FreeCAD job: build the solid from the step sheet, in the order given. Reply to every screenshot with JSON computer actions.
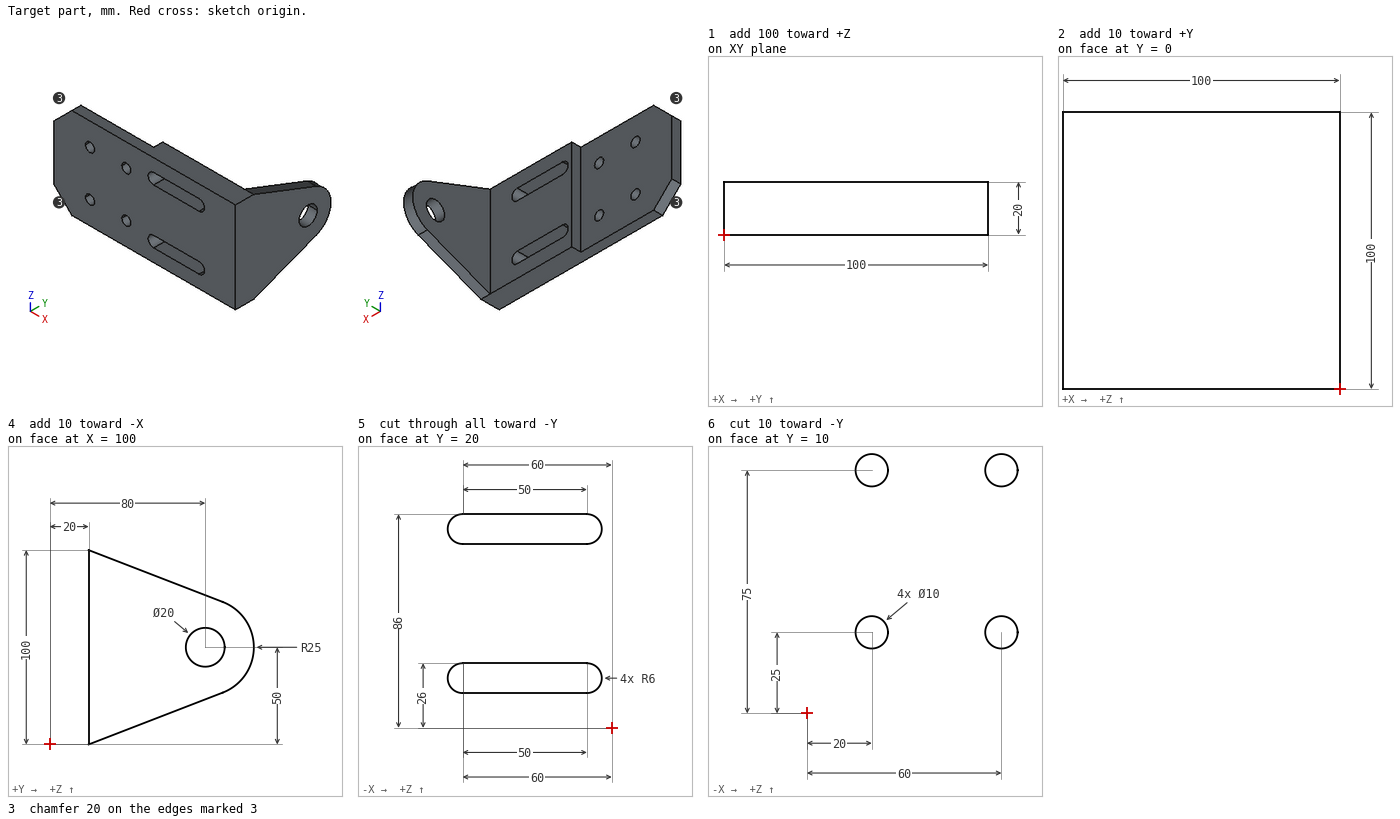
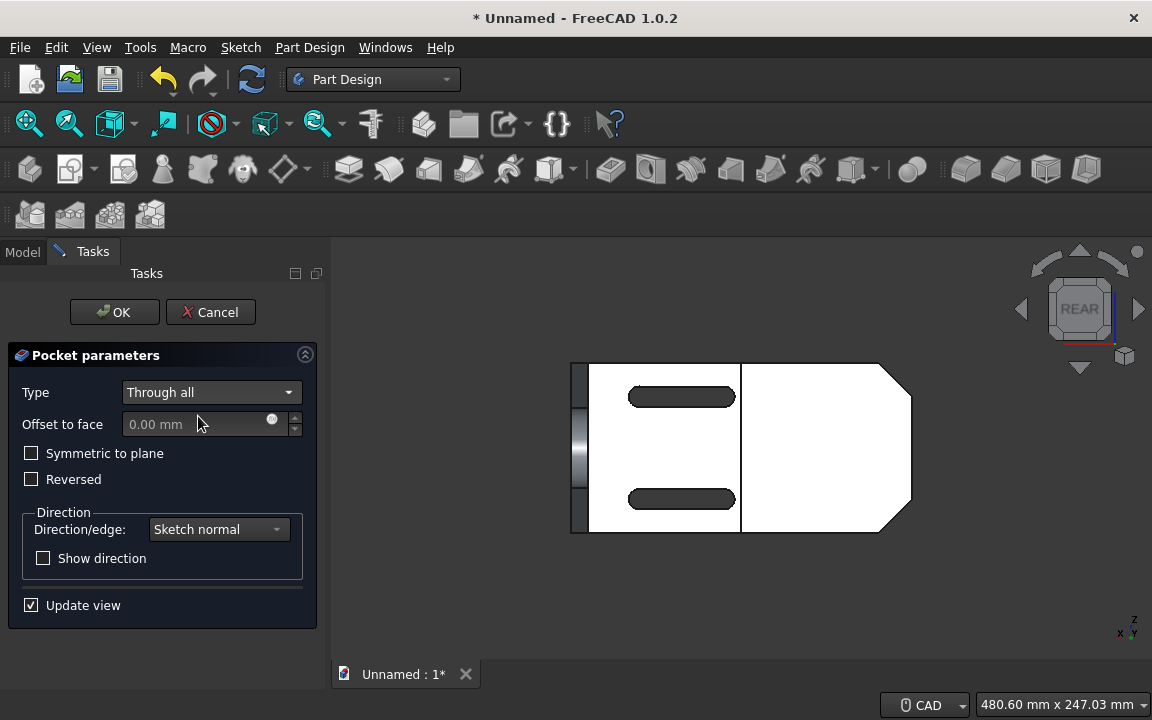
{"action": "left_click", "coordinate": [115, 312]}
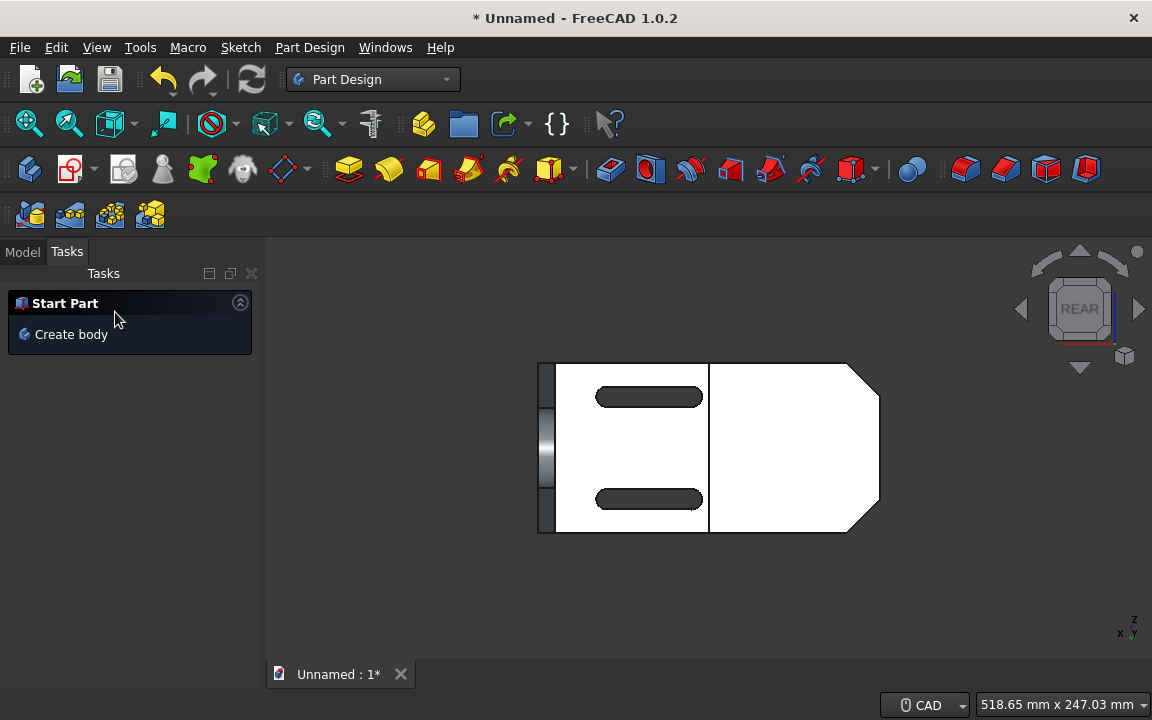
{"action": "left_click", "coordinate": [30, 124]}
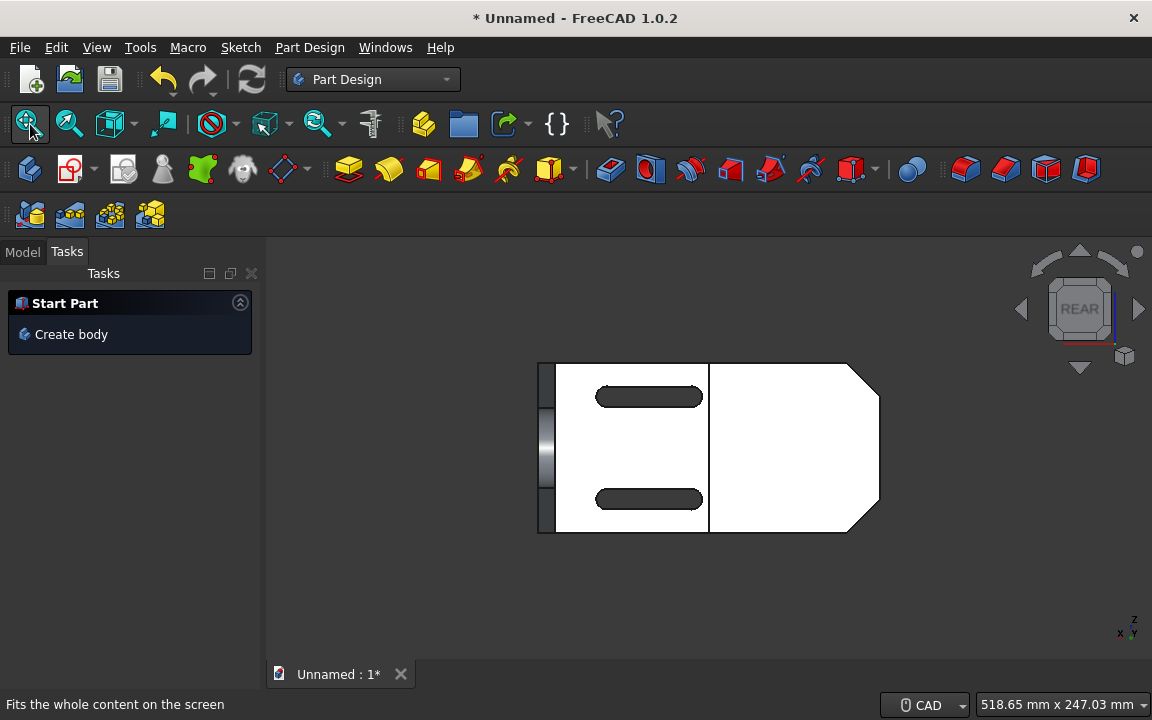
{"action": "left_click", "coordinate": [794, 447]}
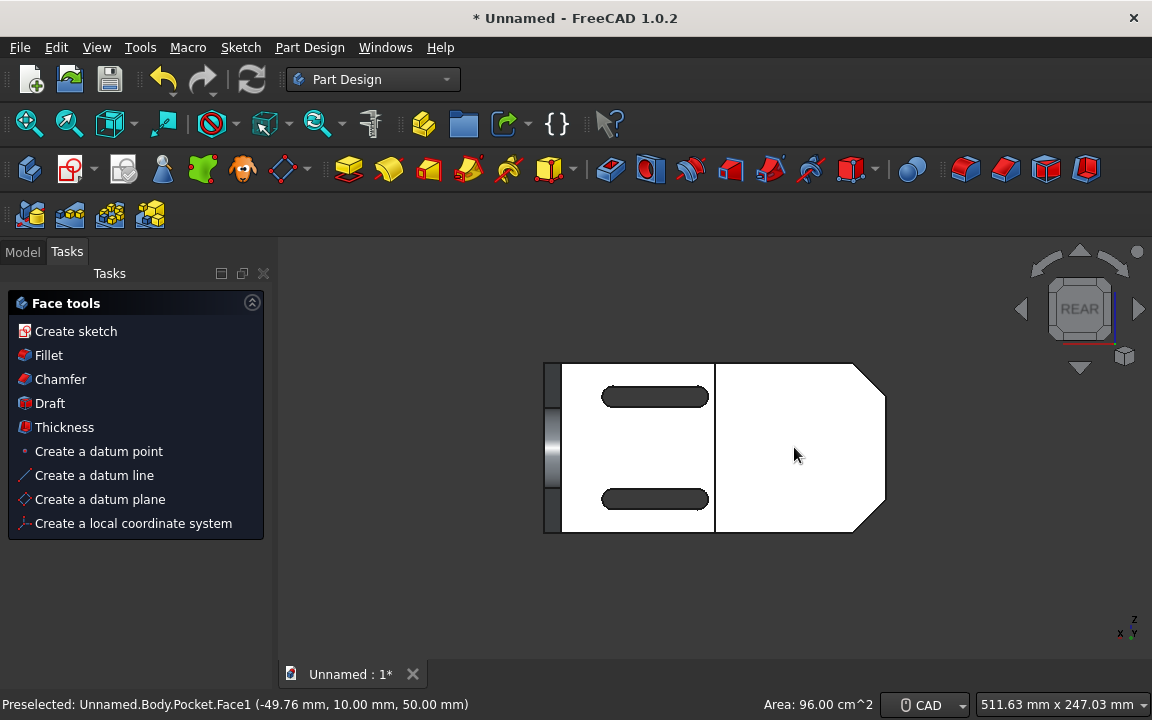
{"action": "left_click", "coordinate": [70, 170]}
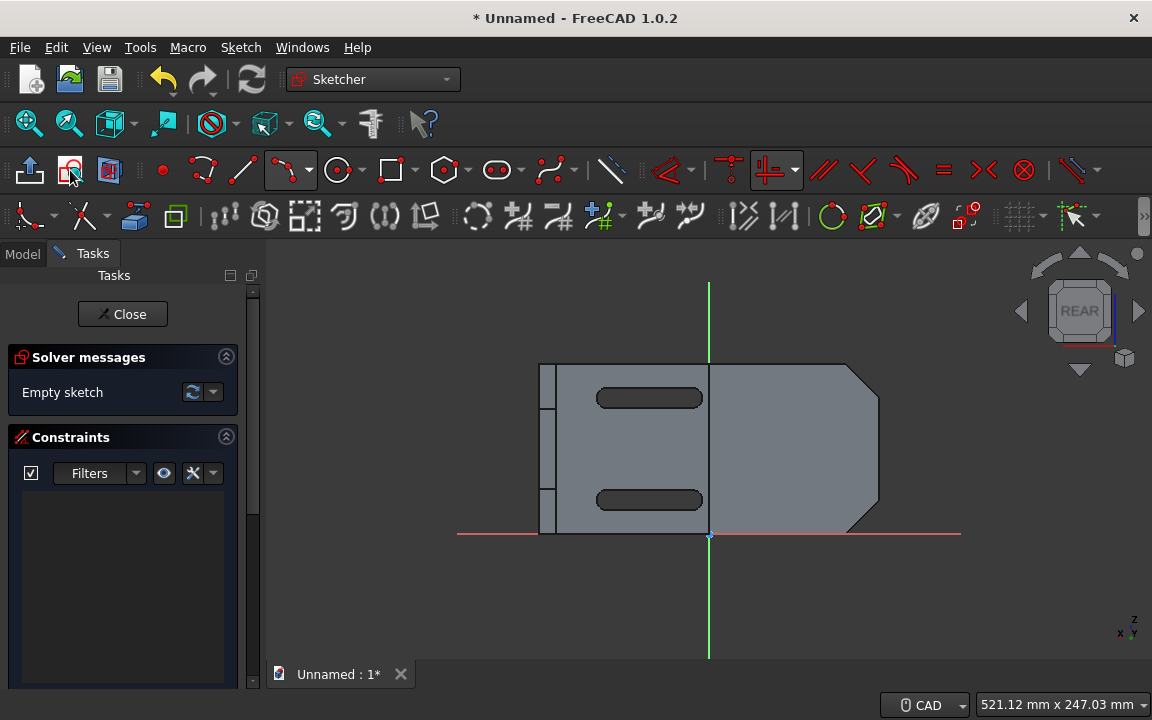
{"action": "scroll", "coordinate": [915, 487], "scroll_direction": "up", "scroll_amount": 3}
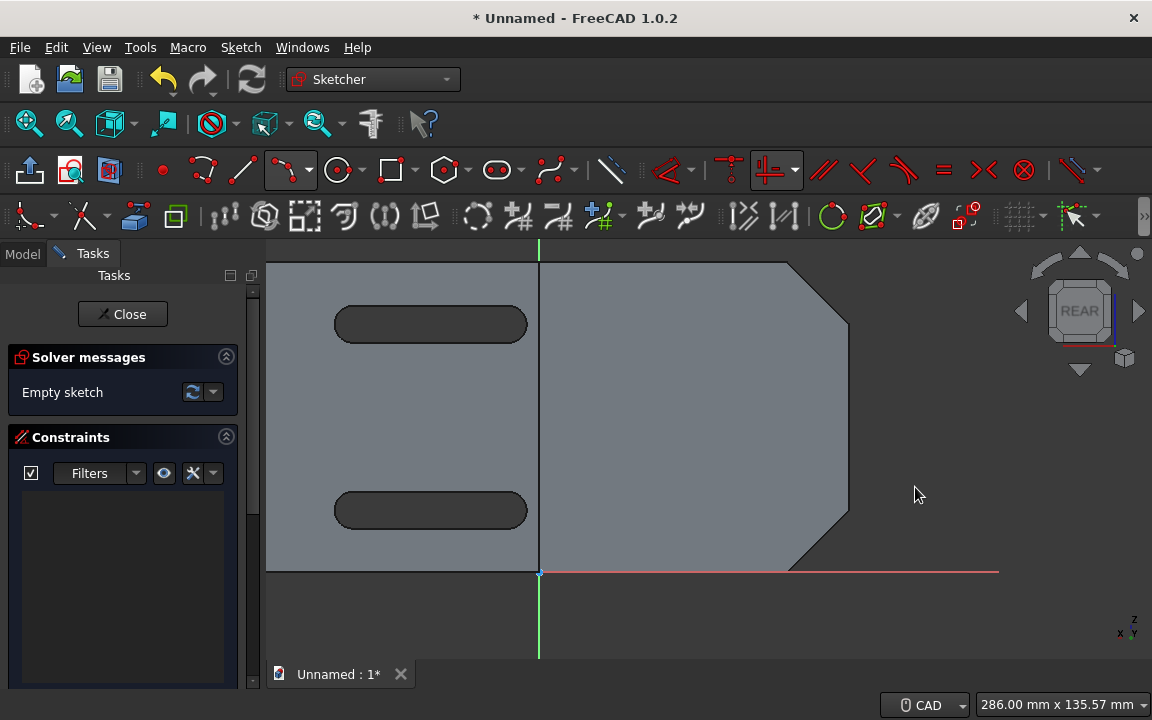
{"action": "left_click", "coordinate": [338, 170]}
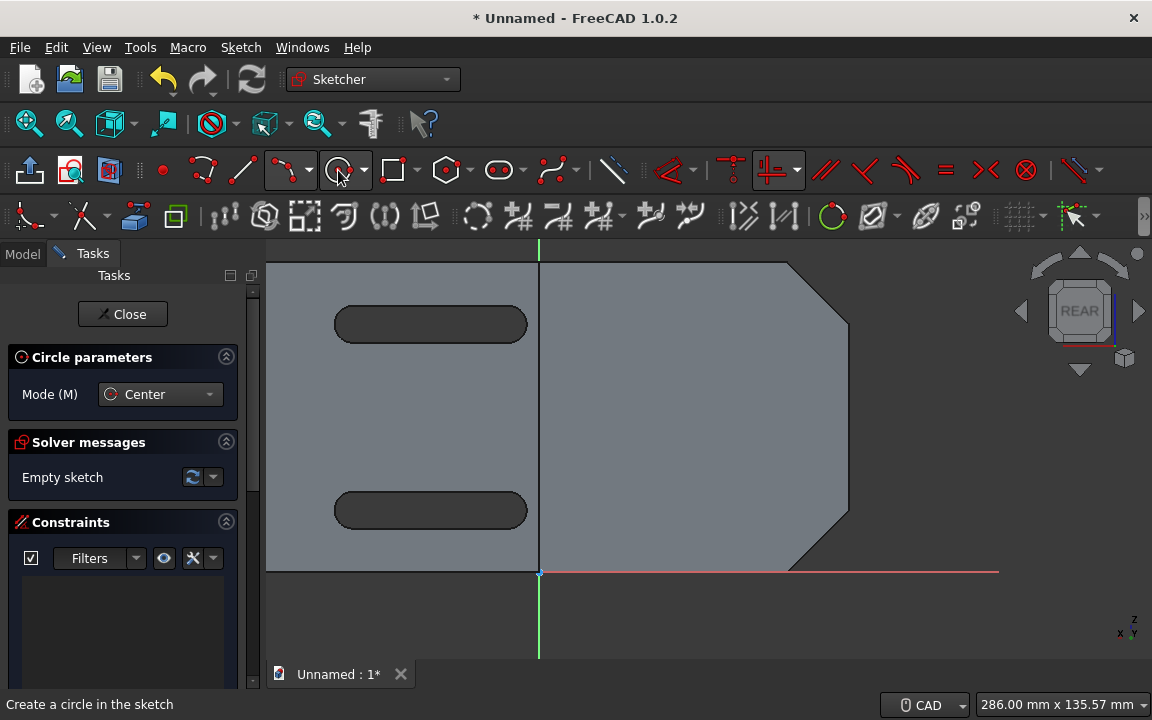
{"action": "scroll", "coordinate": [601, 495], "scroll_direction": "up", "scroll_amount": 2}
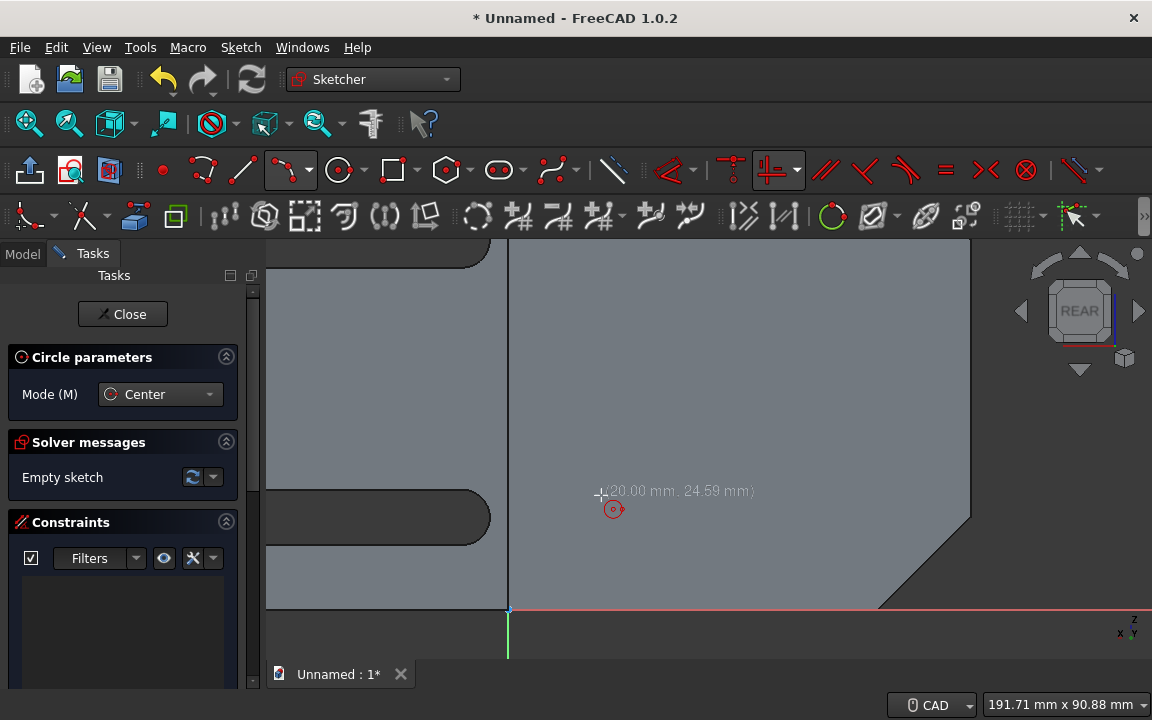
{"action": "left_click", "coordinate": [601, 494]}
{"action": "left_click", "coordinate": [617, 478]}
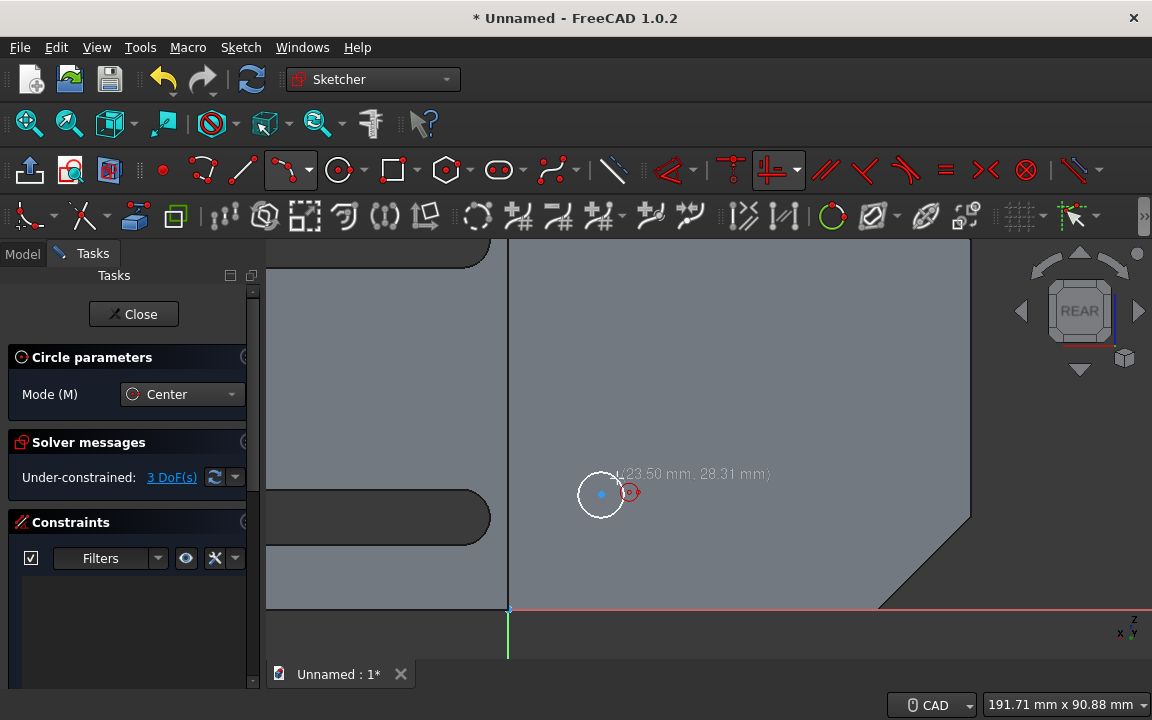
{"action": "left_click", "coordinate": [786, 494]}
{"action": "left_click", "coordinate": [802, 478]}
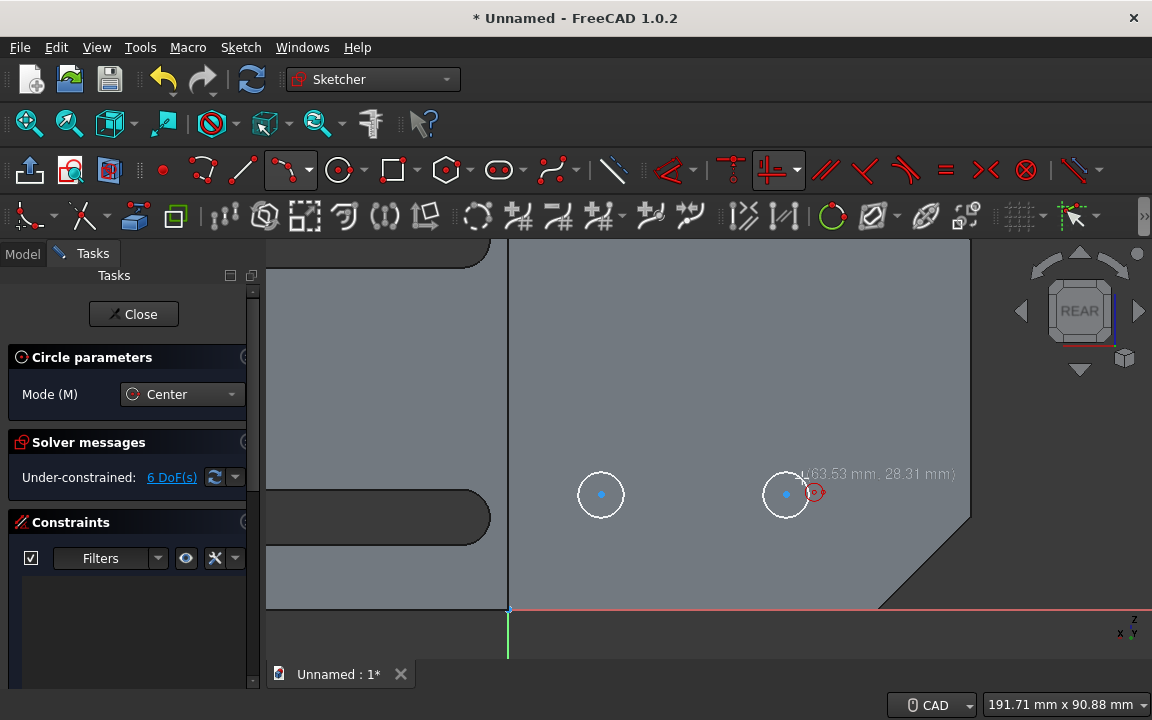
{"action": "scroll", "coordinate": [604, 498], "scroll_direction": "down", "scroll_amount": 2}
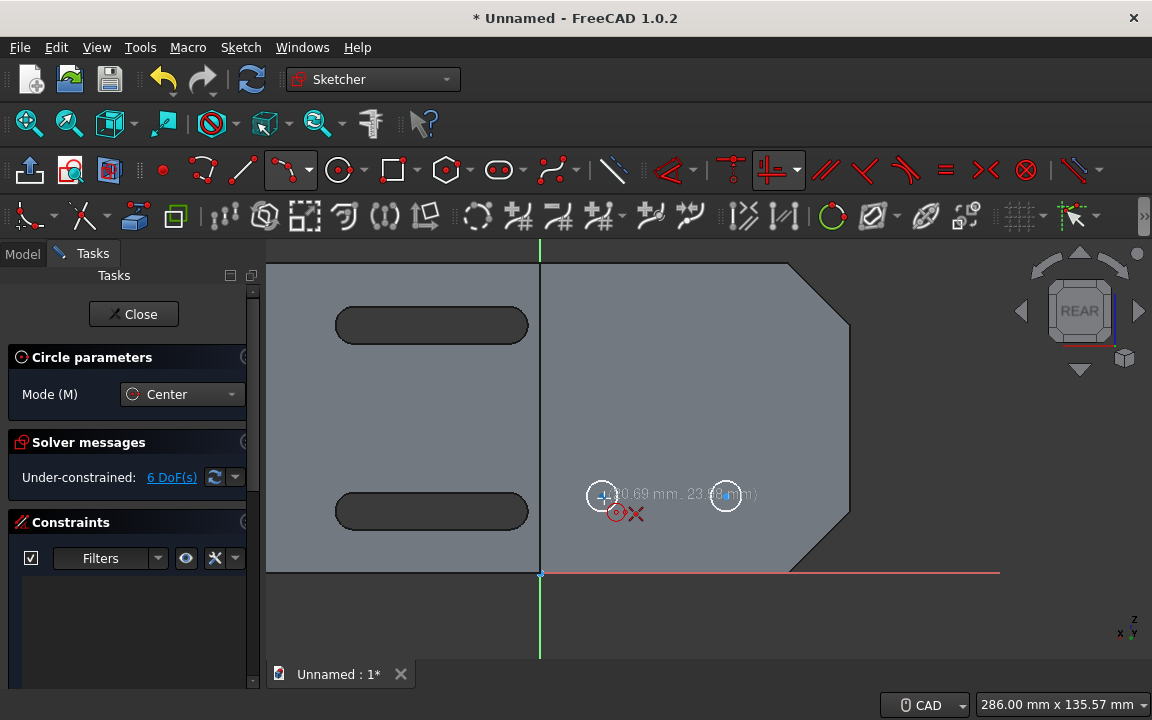
{"action": "scroll", "coordinate": [602, 341], "scroll_direction": "up", "scroll_amount": 2}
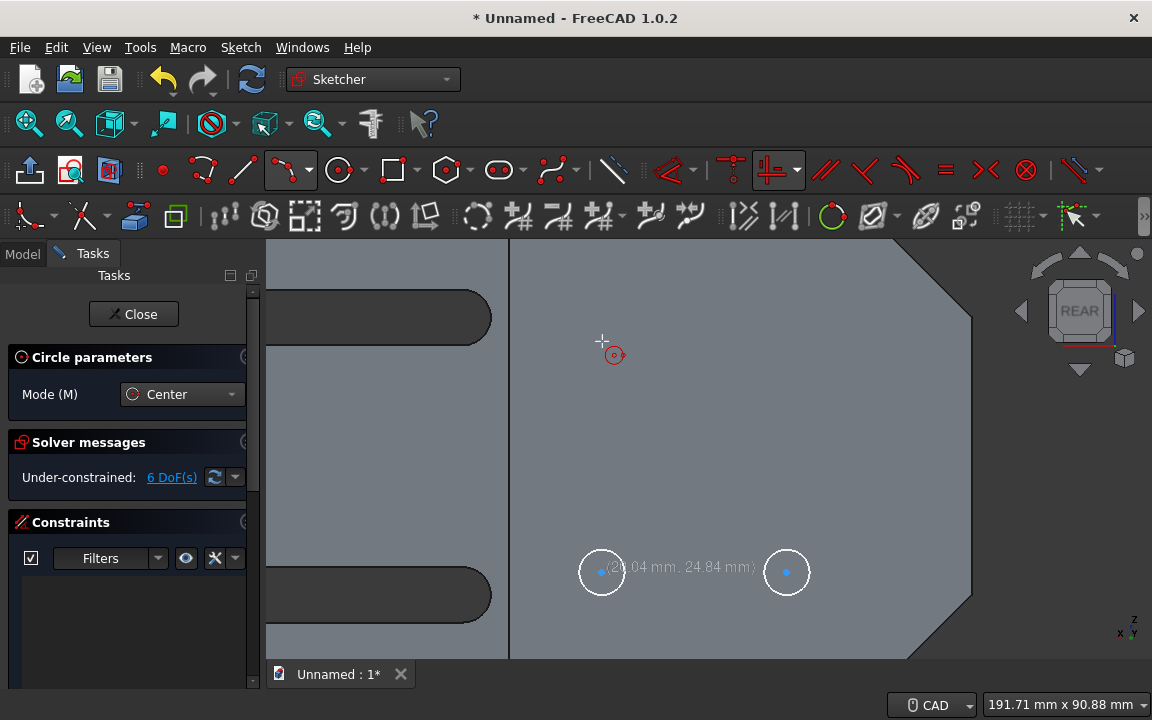
{"action": "left_click", "coordinate": [602, 341]}
{"action": "left_click", "coordinate": [618, 324]}